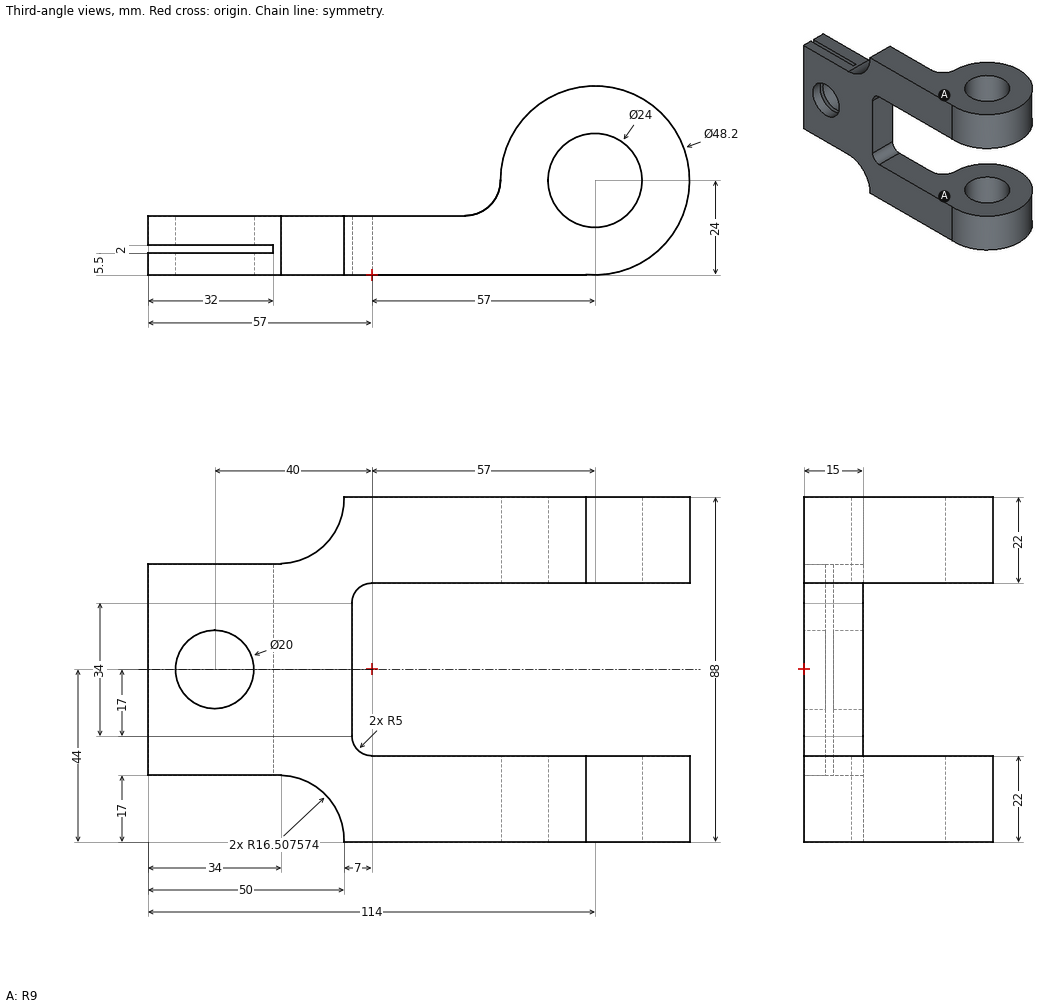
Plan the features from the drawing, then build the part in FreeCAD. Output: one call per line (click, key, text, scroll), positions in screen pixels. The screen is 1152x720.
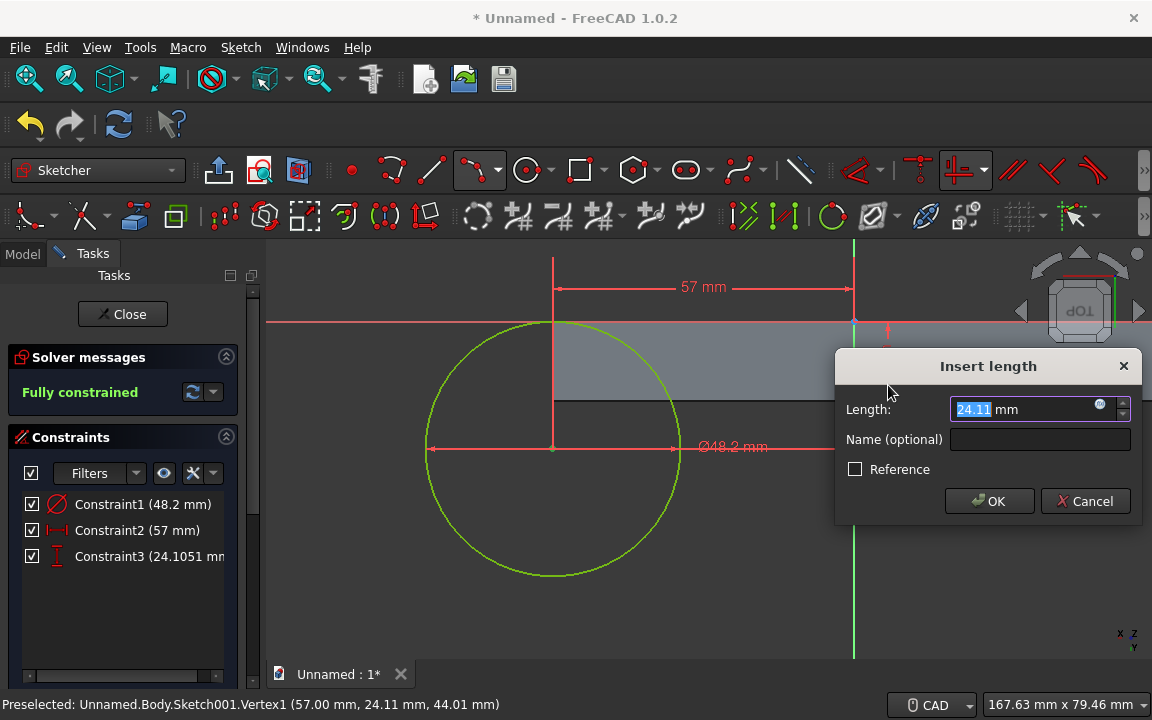
text(24)
key(Return)
key(Escape)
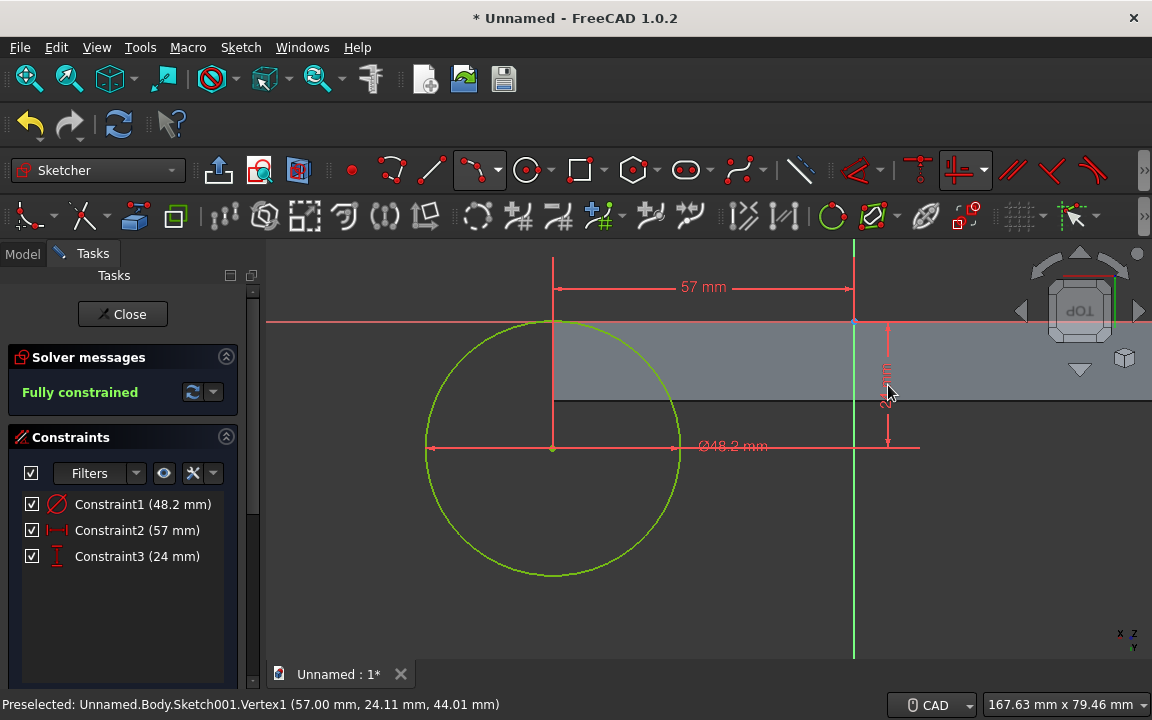
click(123, 314)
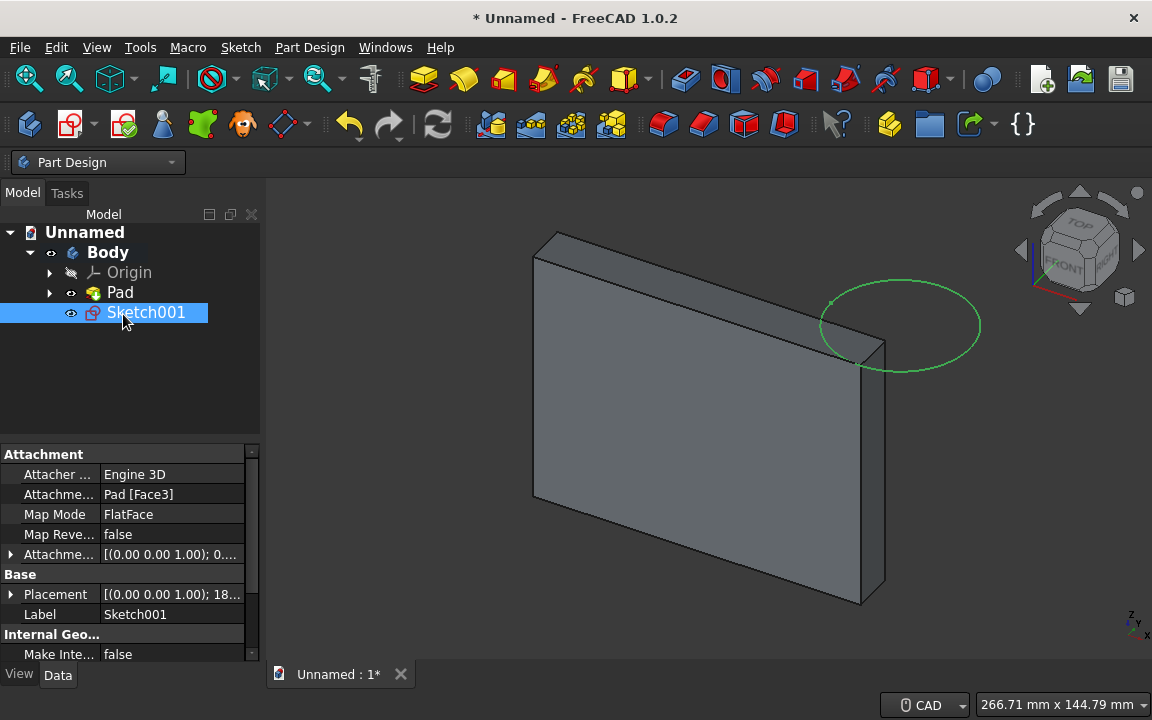
click(424, 80)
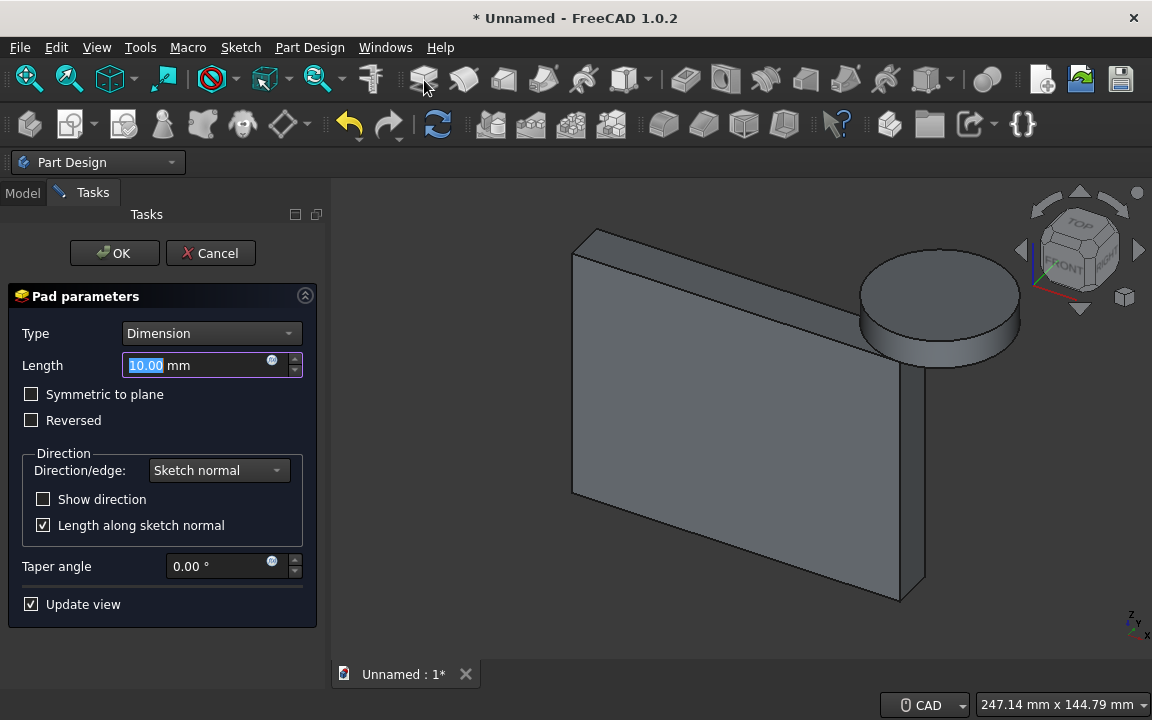
text(22)
key(Tab)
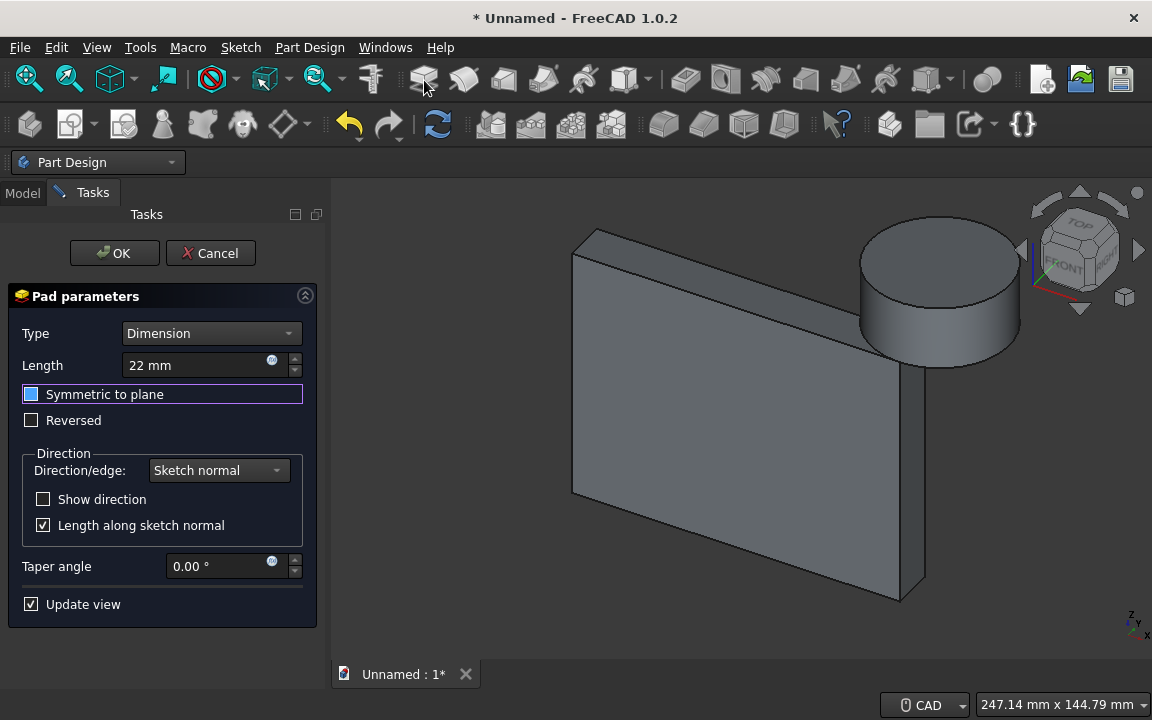
click(30, 420)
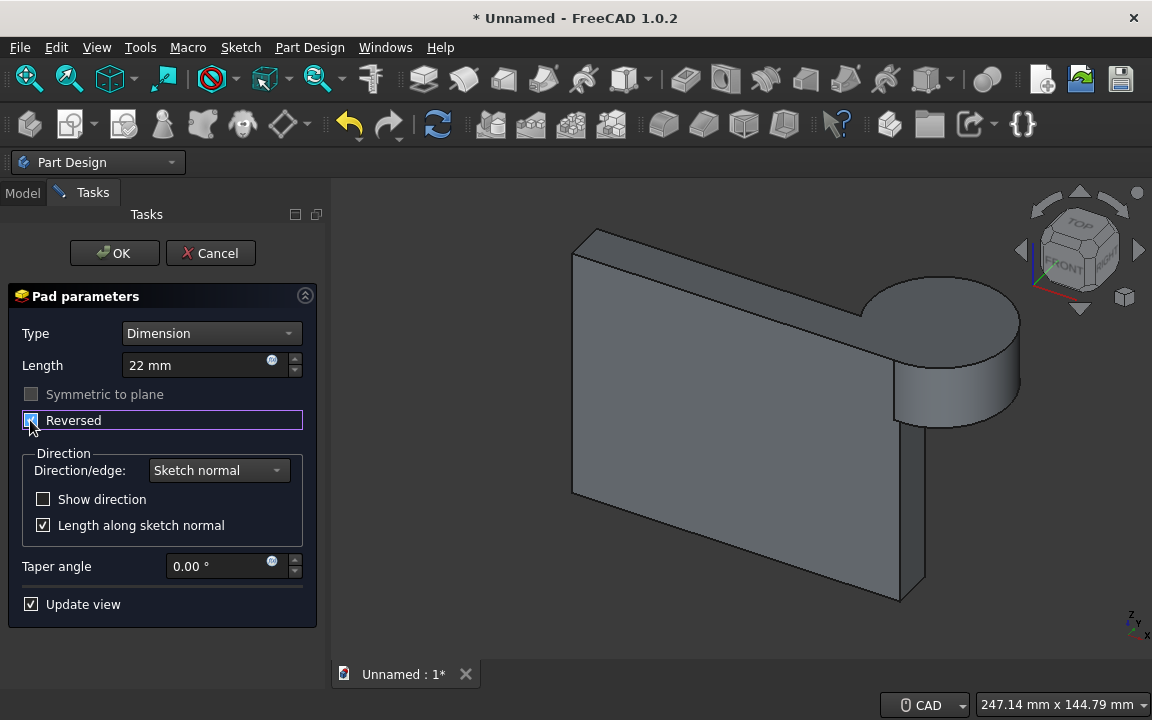
click(115, 253)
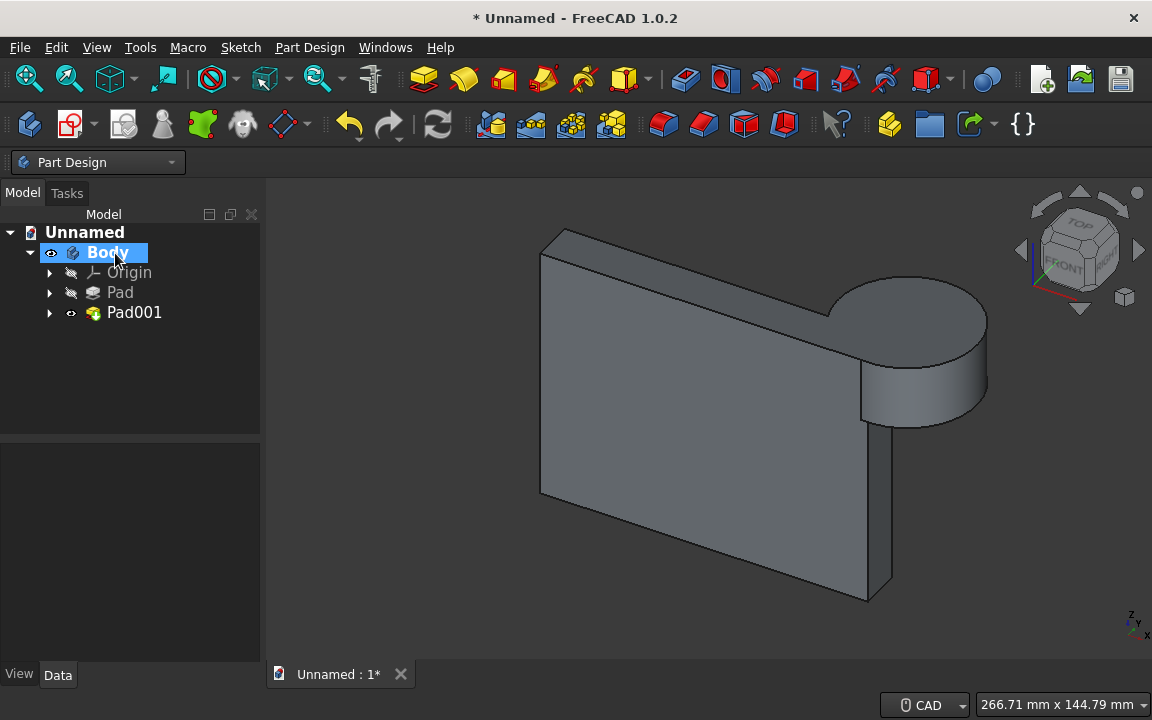
key(v)
key(f)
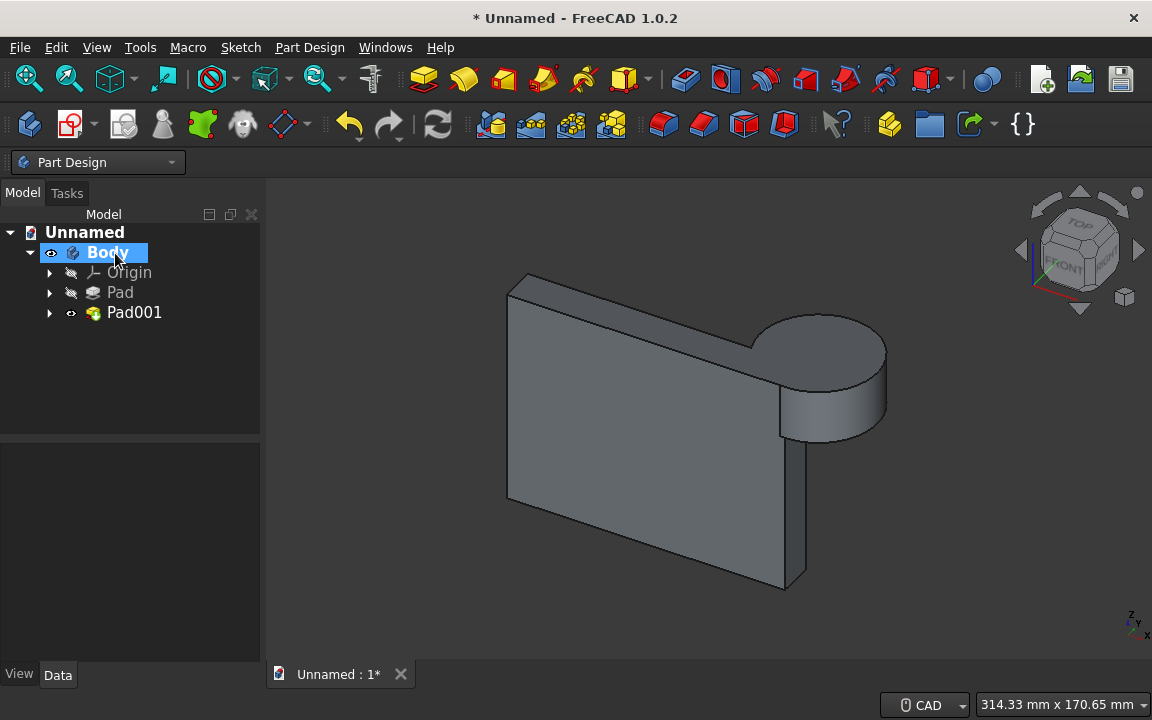
click(50, 273)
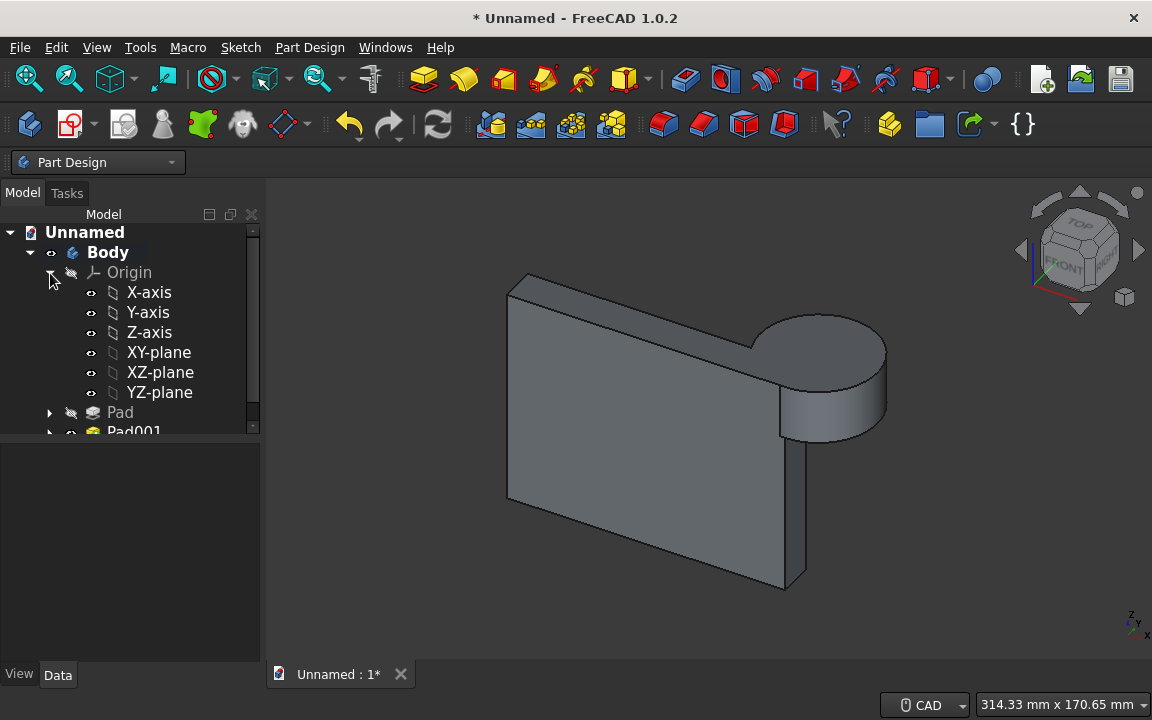
click(136, 353)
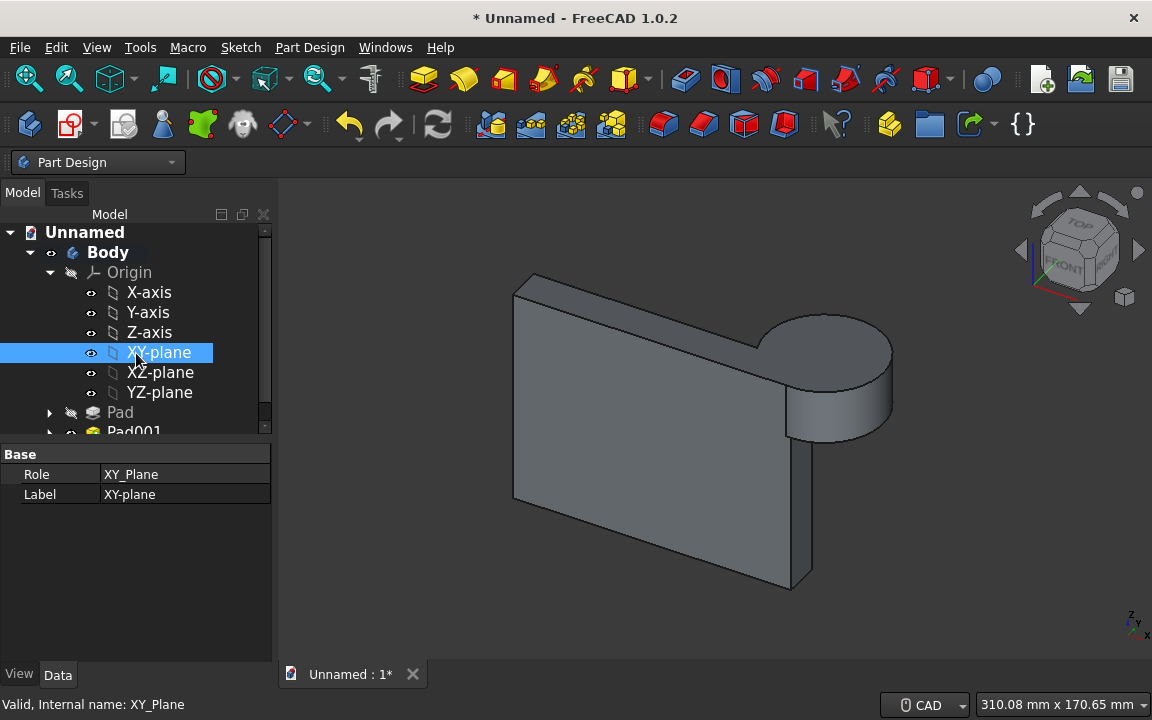
click(284, 124)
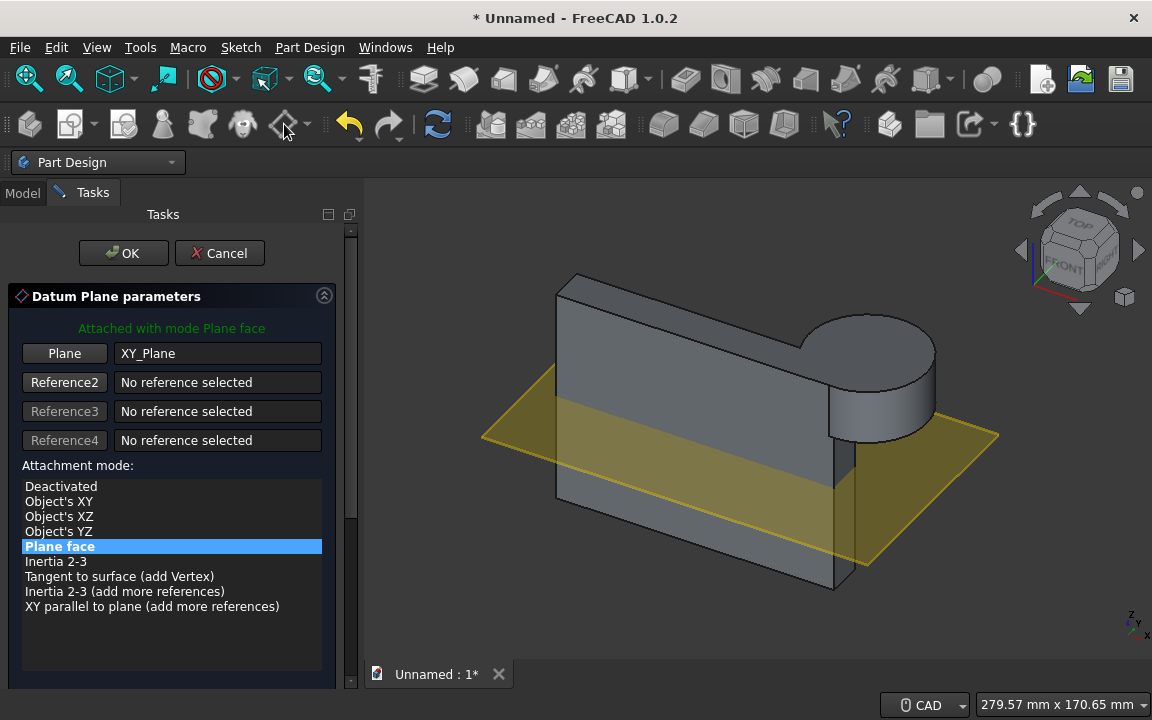
scroll(351, 456, down, 3)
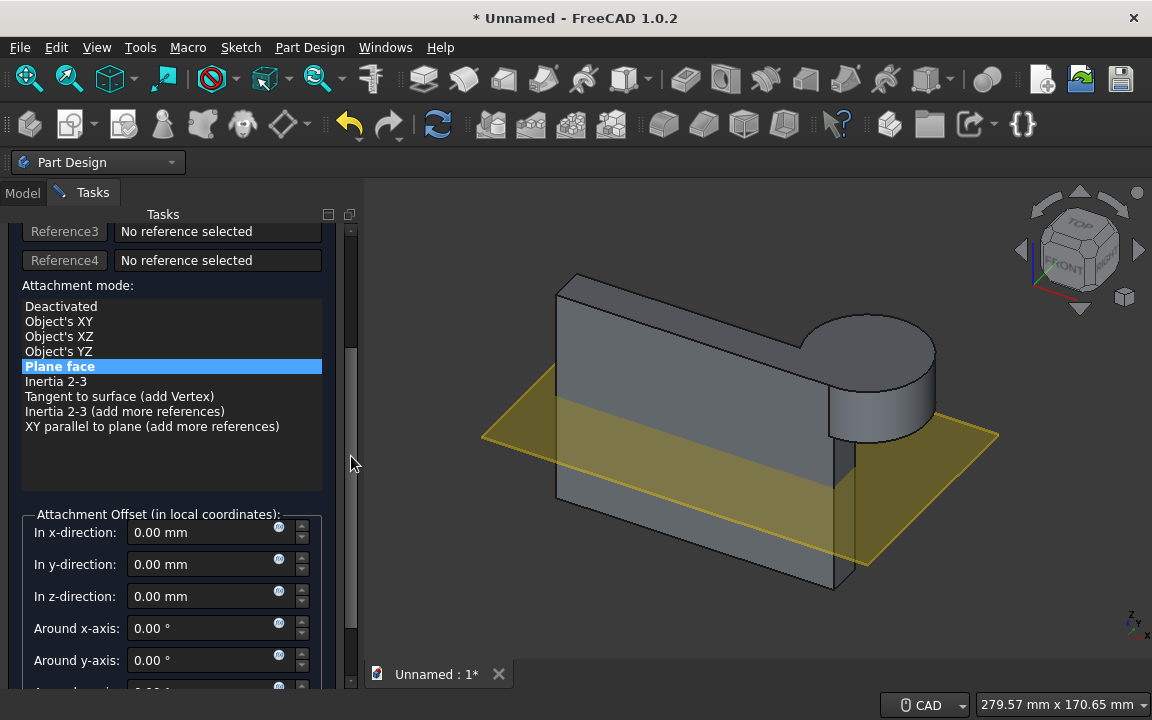
triple_click(210, 596)